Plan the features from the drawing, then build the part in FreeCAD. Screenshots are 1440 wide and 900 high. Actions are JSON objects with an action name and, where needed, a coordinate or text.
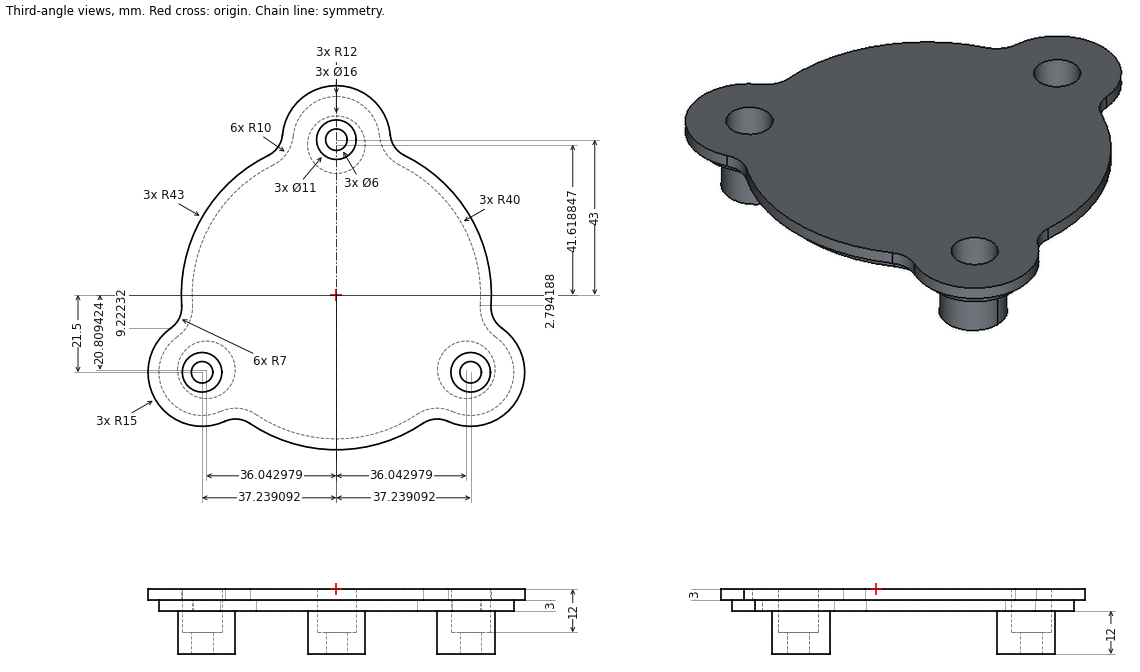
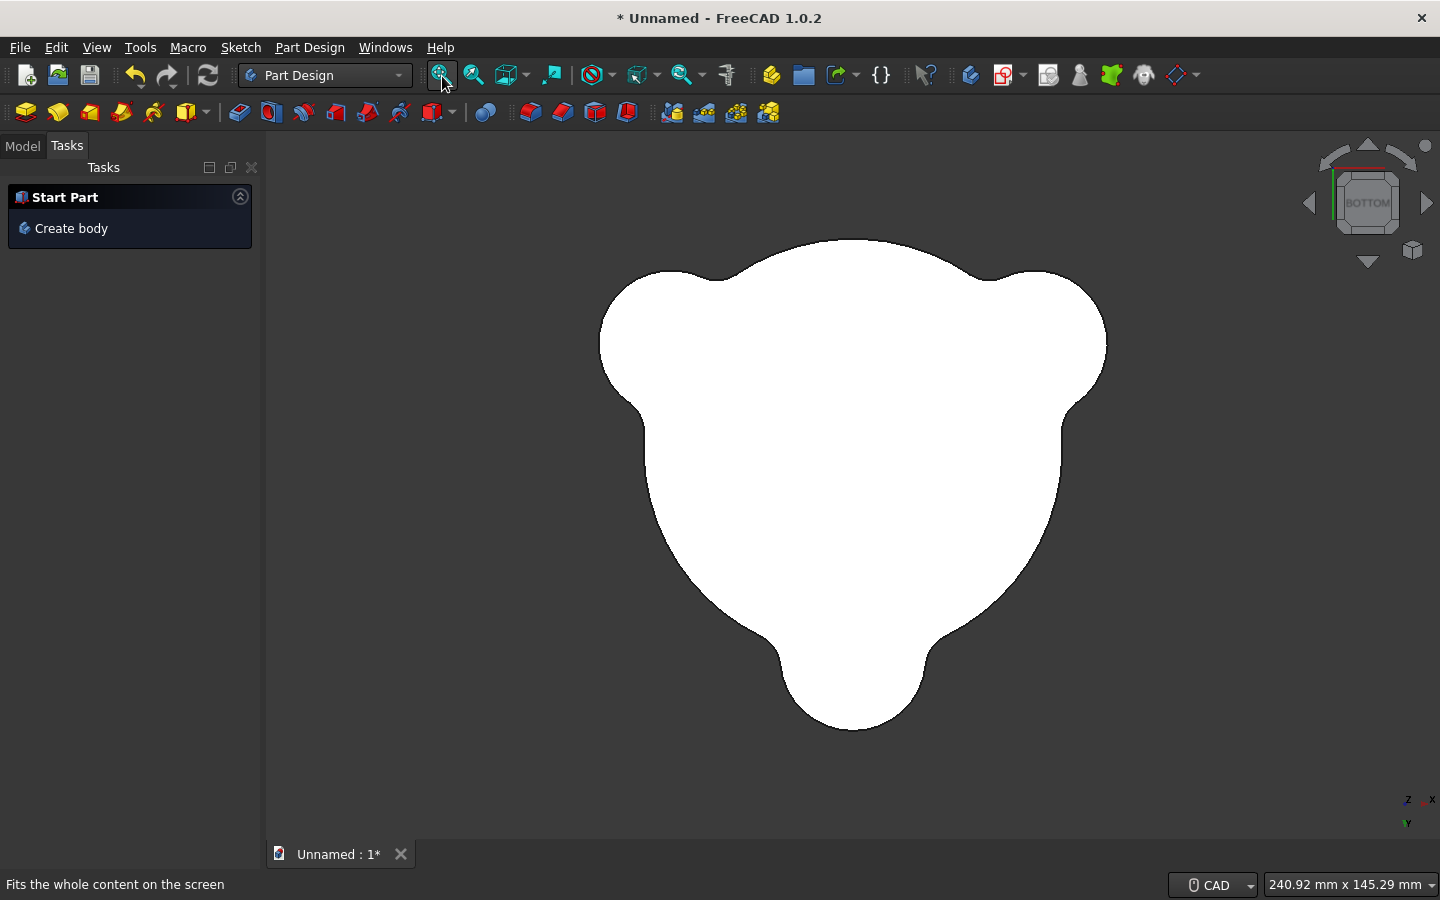
{"action": "left_click", "coordinate": [853, 484]}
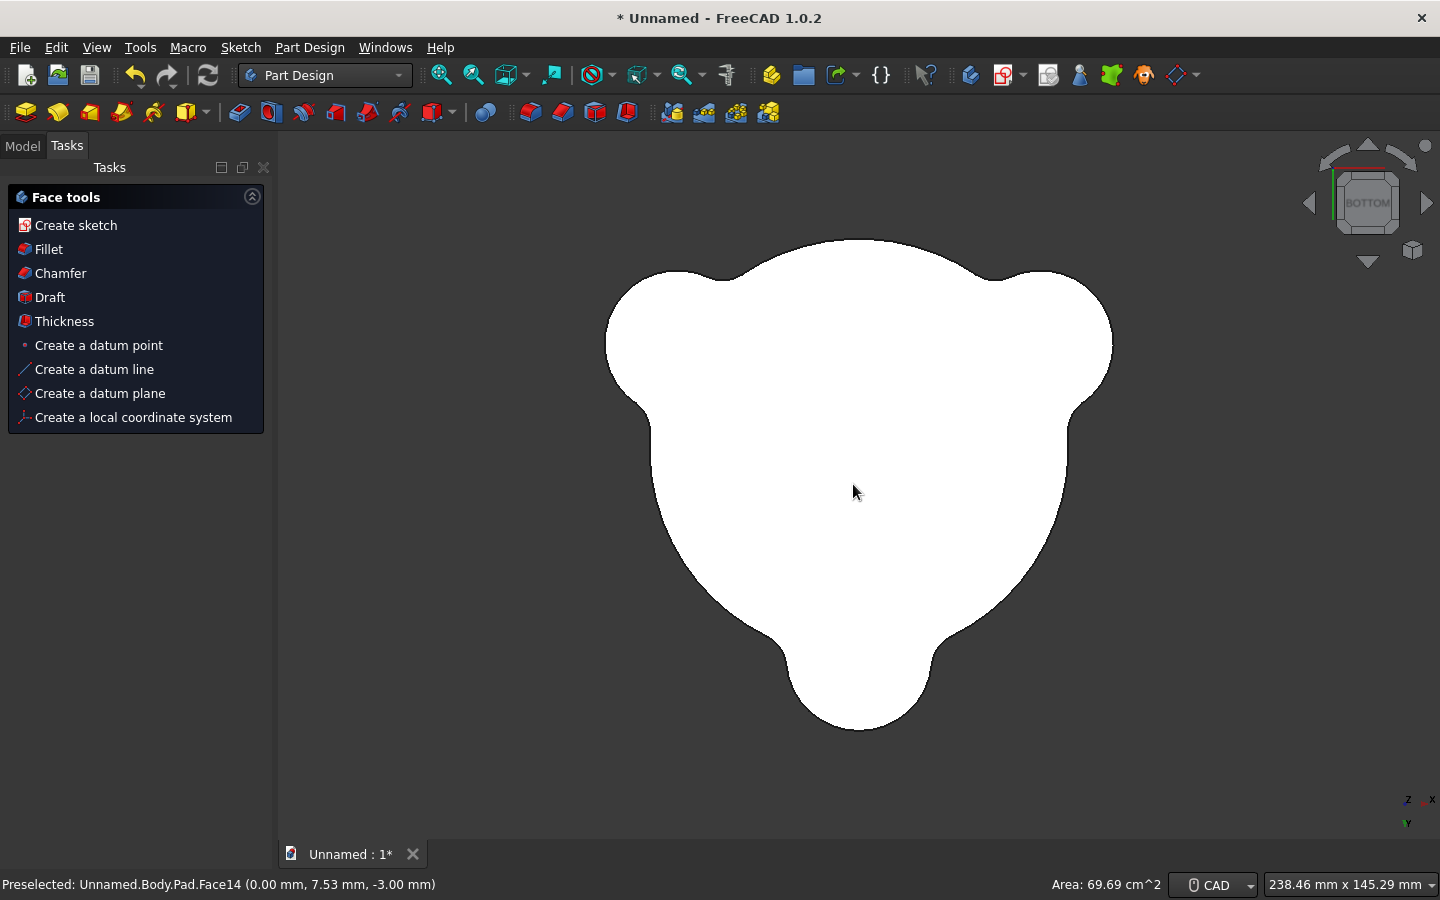
{"action": "left_click", "coordinate": [1004, 76]}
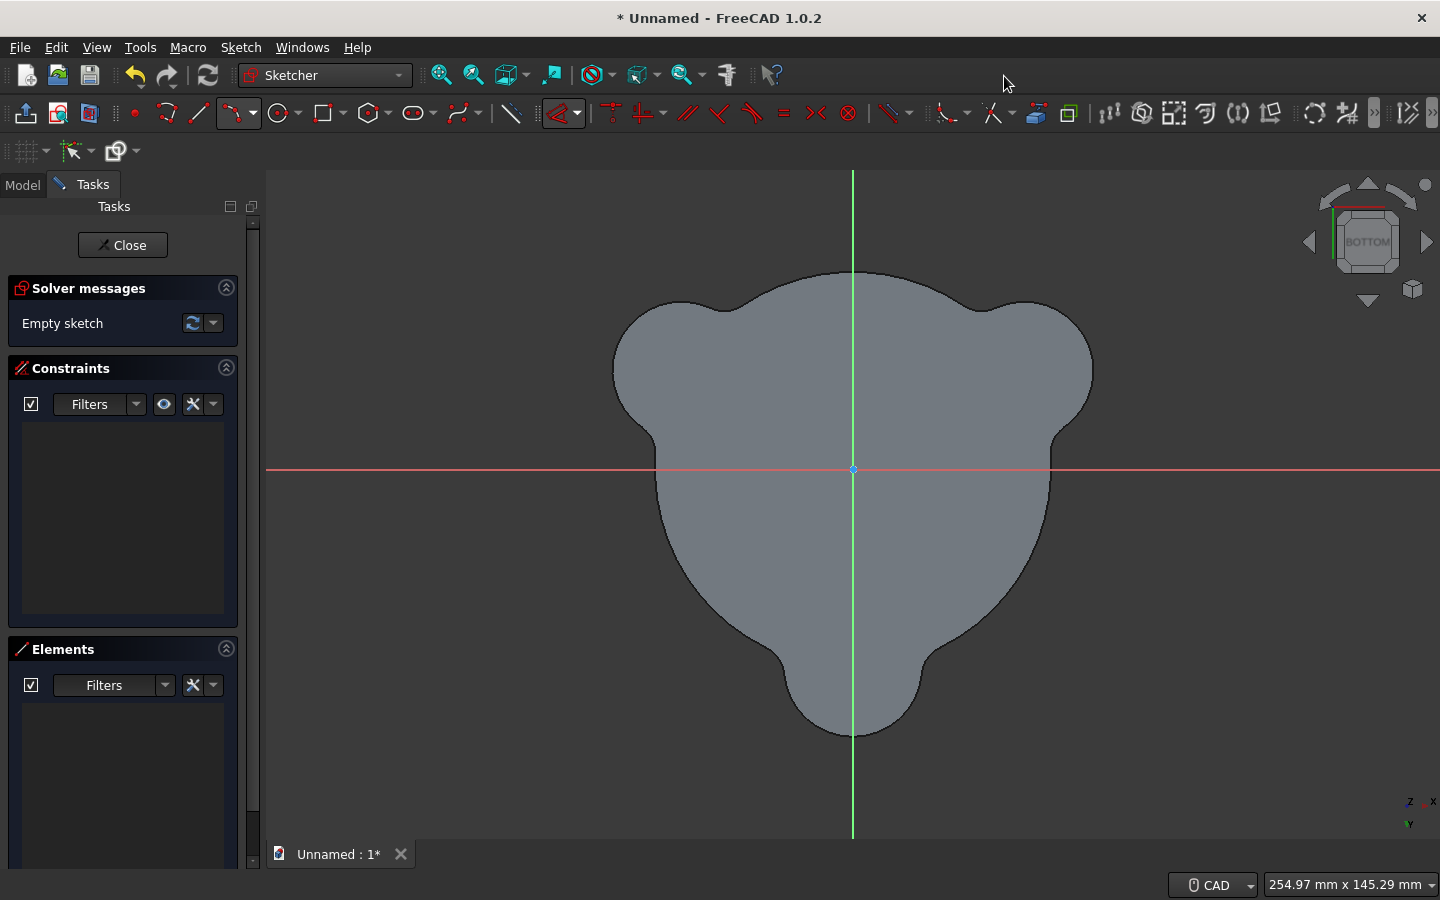
{"action": "left_click", "coordinate": [232, 114]}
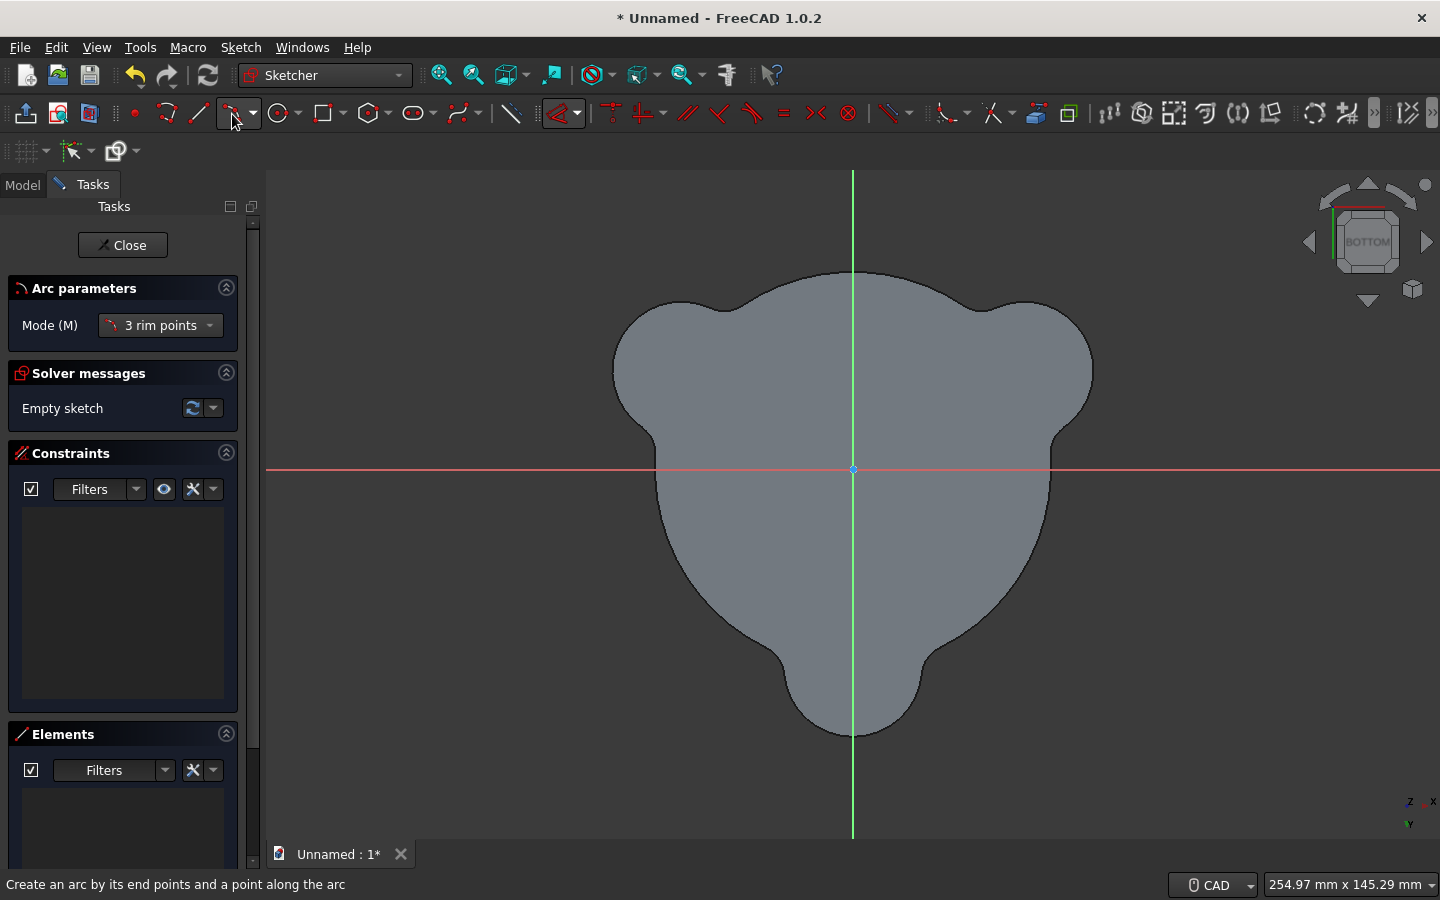
{"action": "left_click", "coordinate": [772, 635]}
{"action": "left_click", "coordinate": [798, 673]}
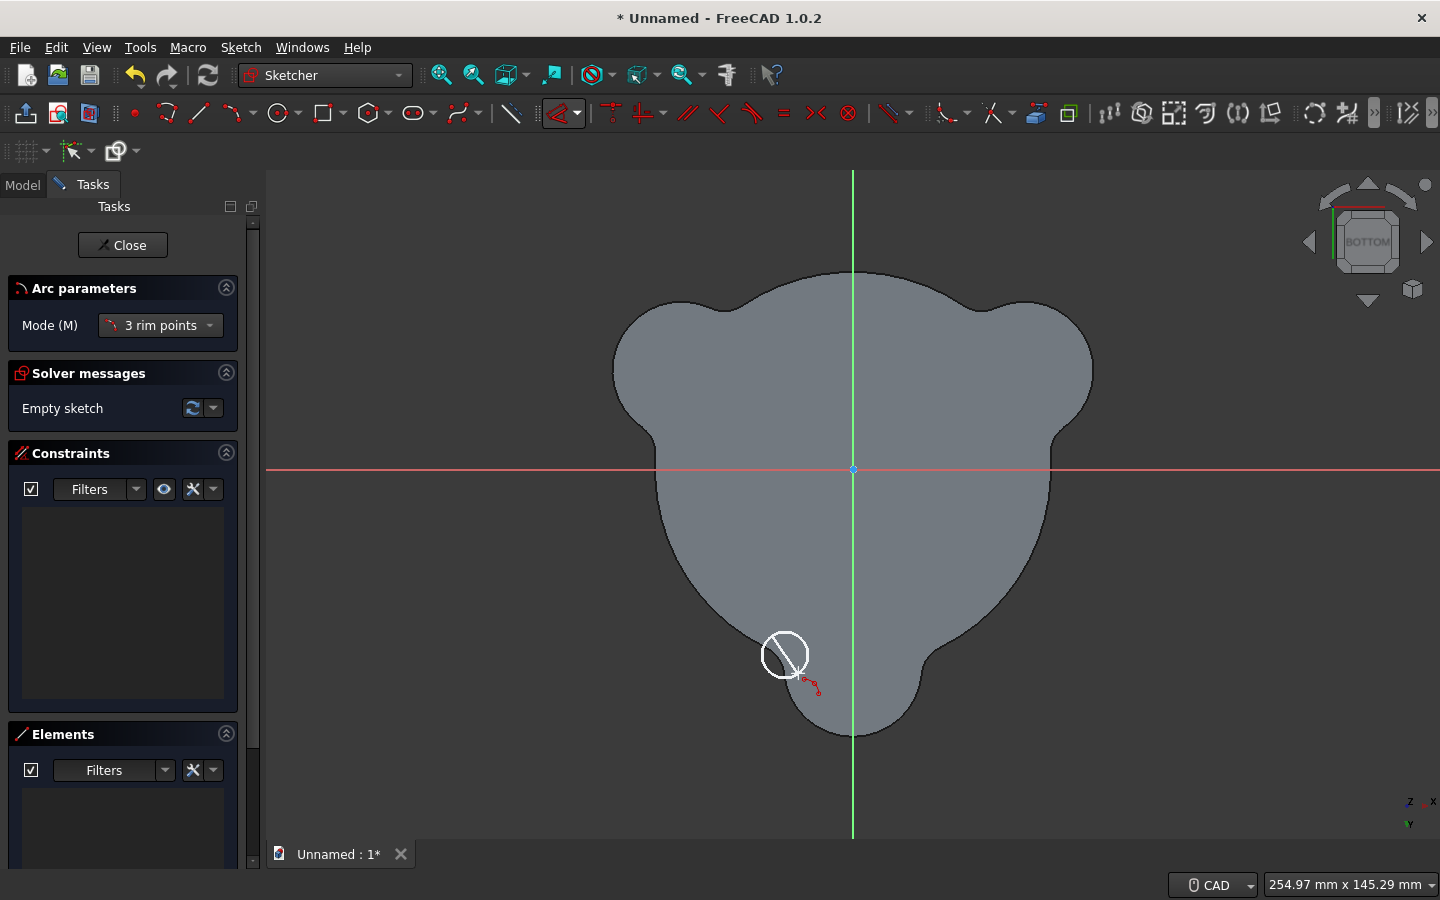
{"action": "scroll", "coordinate": [790, 651], "scroll_direction": "up", "scroll_amount": 5}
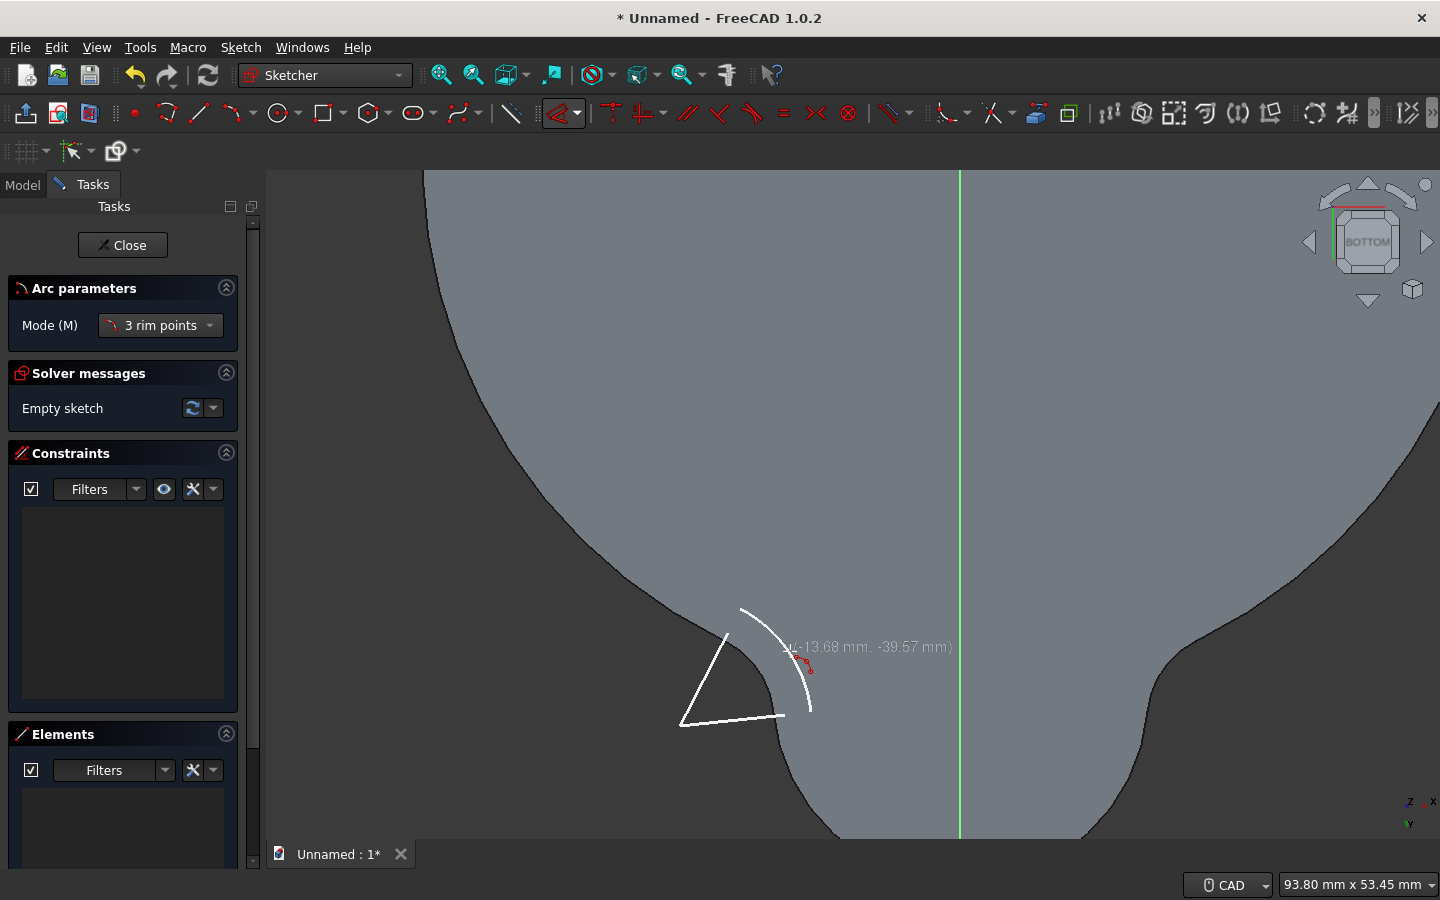
{"action": "left_click", "coordinate": [789, 649]}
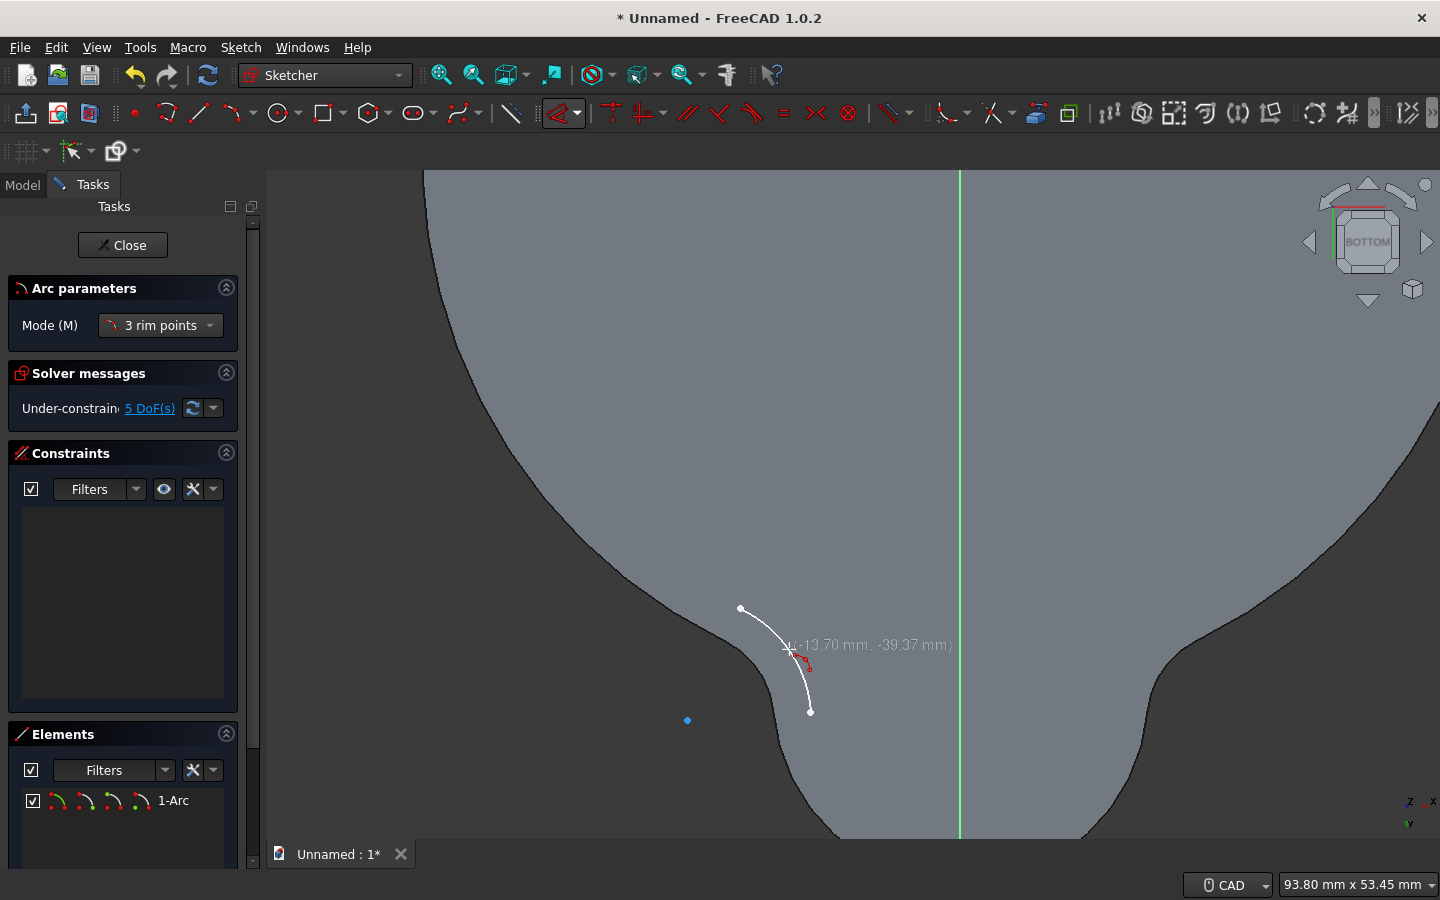
{"action": "left_click", "coordinate": [811, 712]}
{"action": "left_click", "coordinate": [1110, 709]}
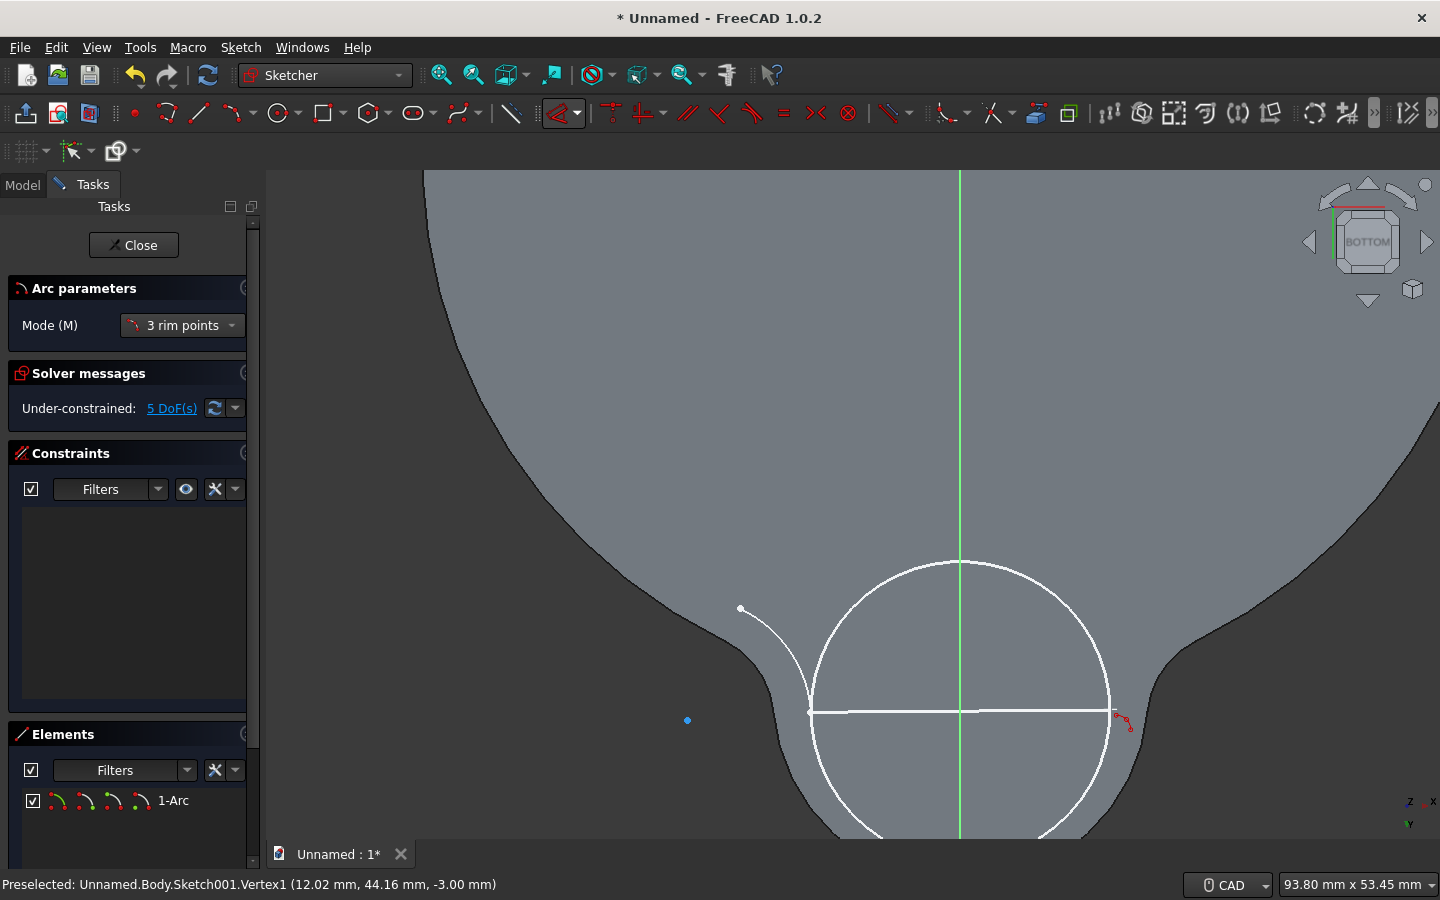
{"action": "scroll", "coordinate": [682, 652], "scroll_direction": "down", "scroll_amount": 5}